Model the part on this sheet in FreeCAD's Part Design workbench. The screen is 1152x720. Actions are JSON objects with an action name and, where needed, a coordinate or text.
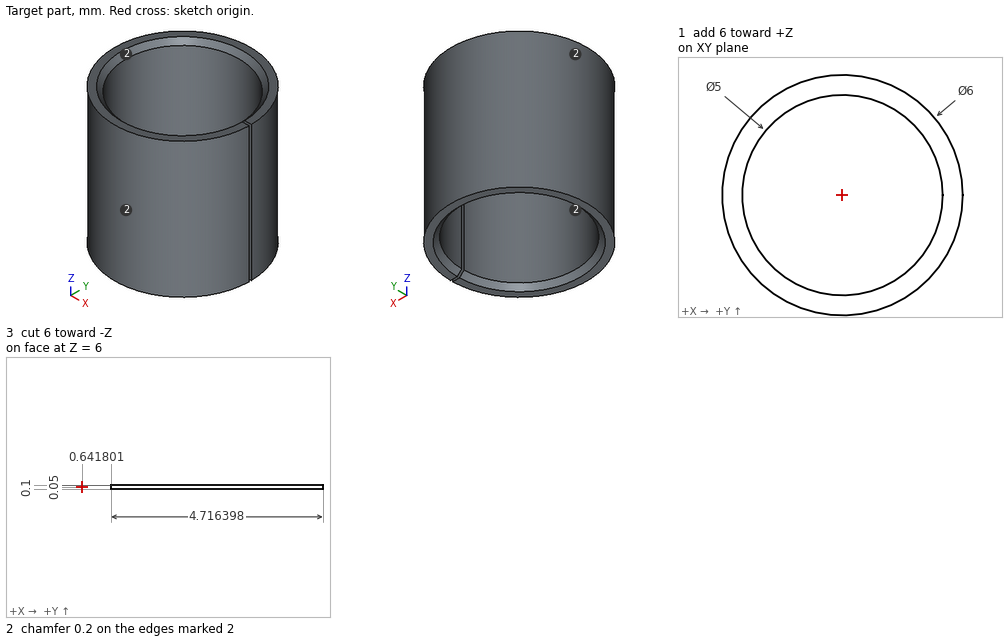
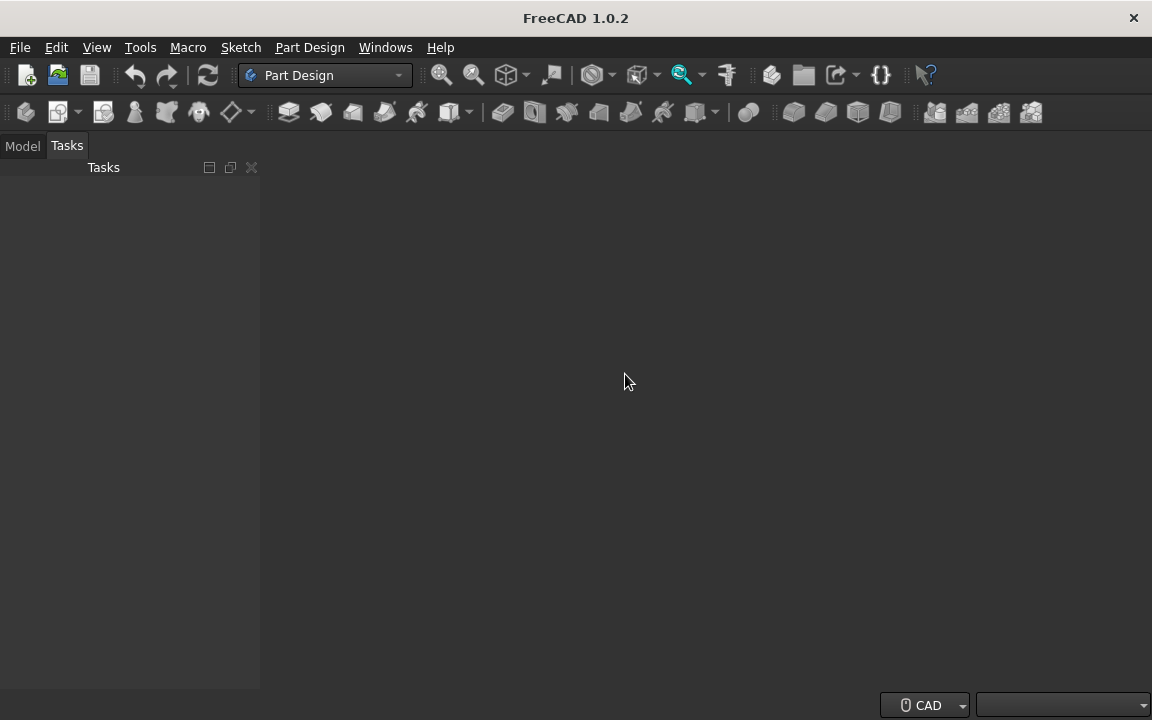
{"action": "left_click", "coordinate": [26, 76]}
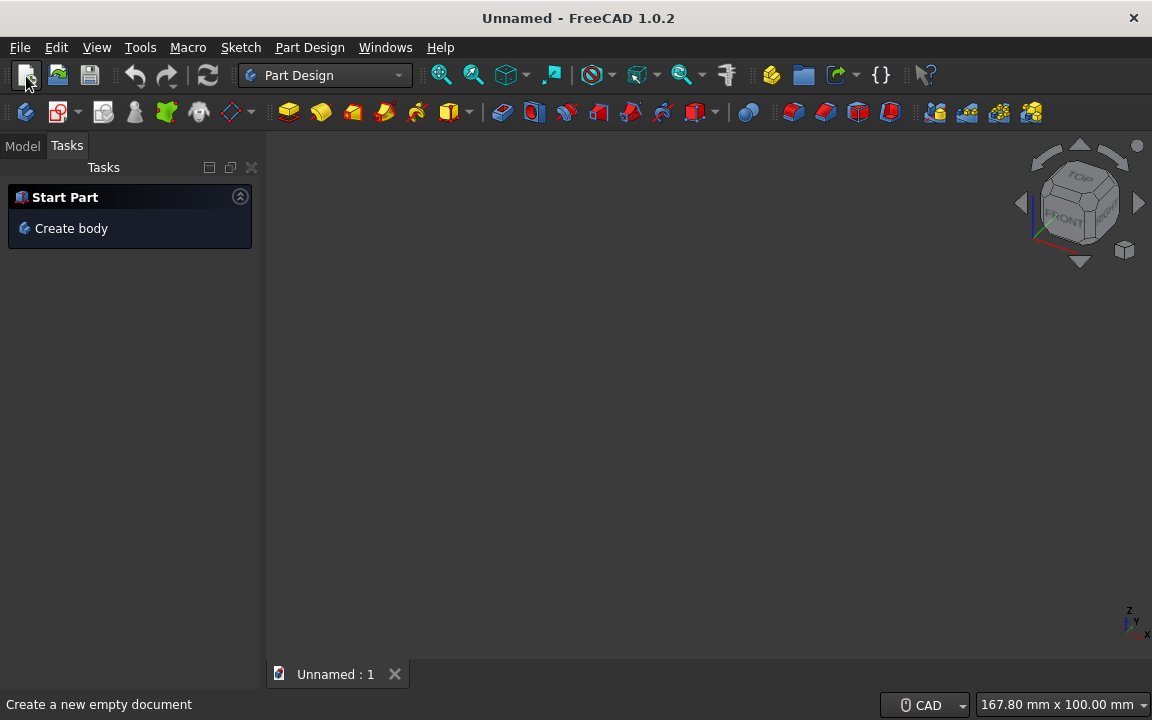
{"action": "left_click", "coordinate": [58, 112]}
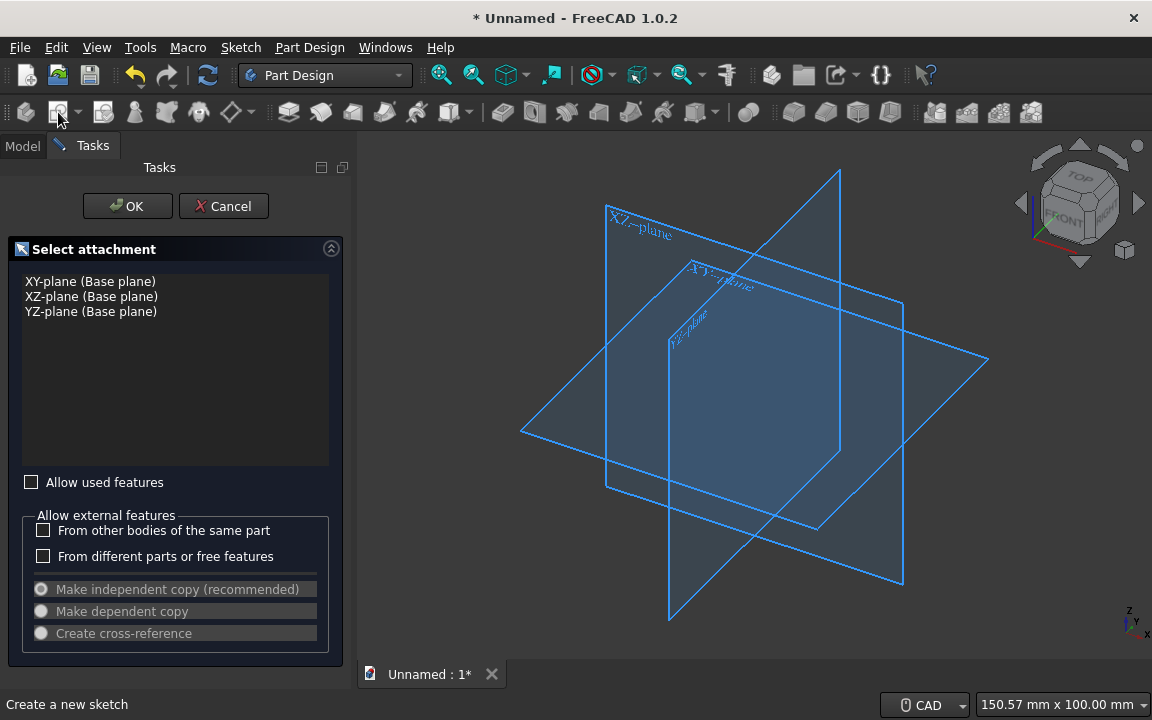
{"action": "left_click", "coordinate": [82, 282]}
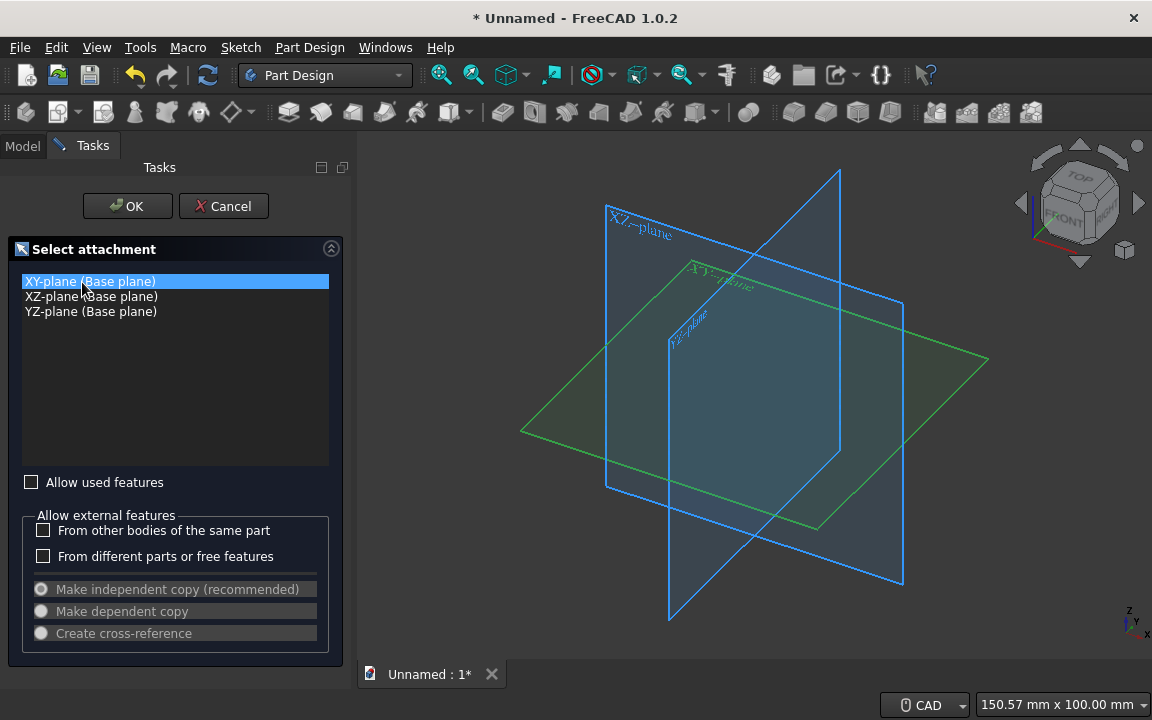
{"action": "left_click", "coordinate": [128, 206]}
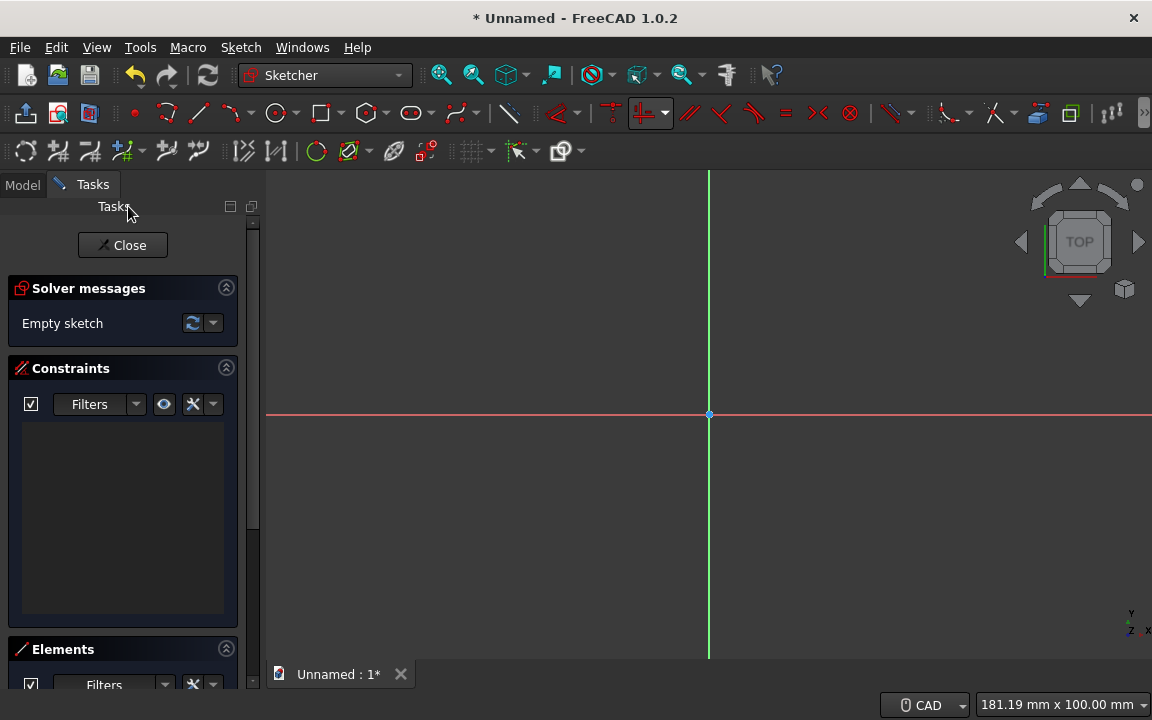
{"action": "scroll", "coordinate": [716, 414], "scroll_direction": "up", "scroll_amount": 12}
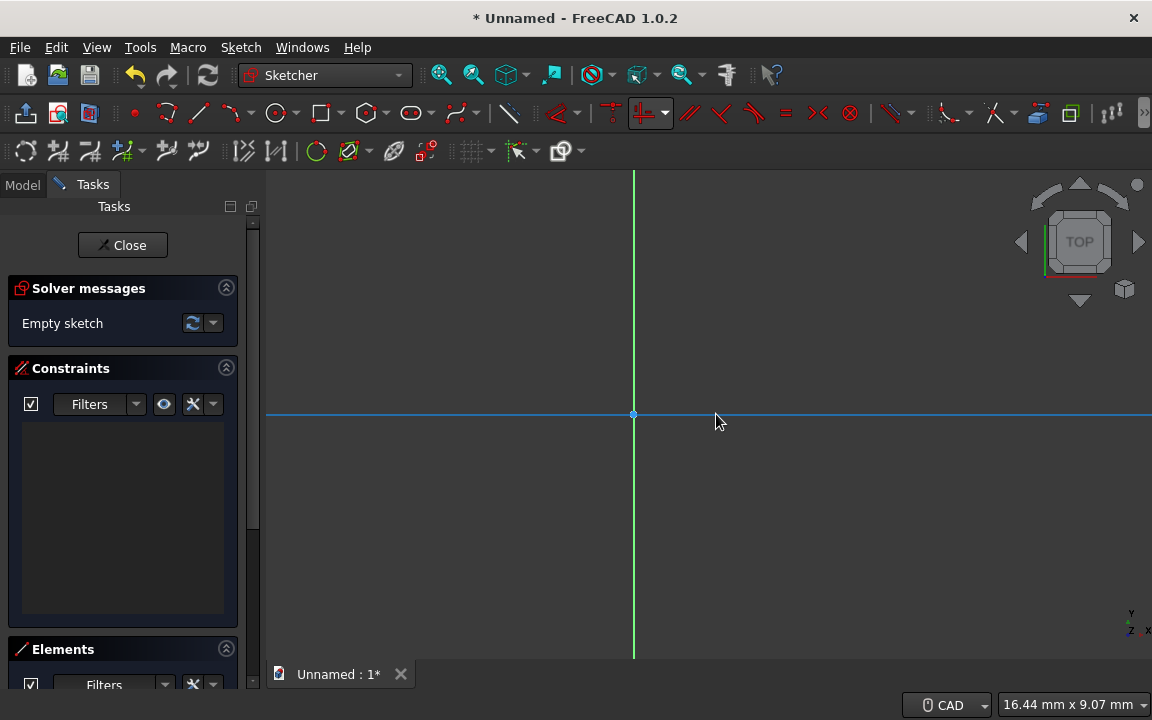
{"action": "left_click", "coordinate": [276, 114]}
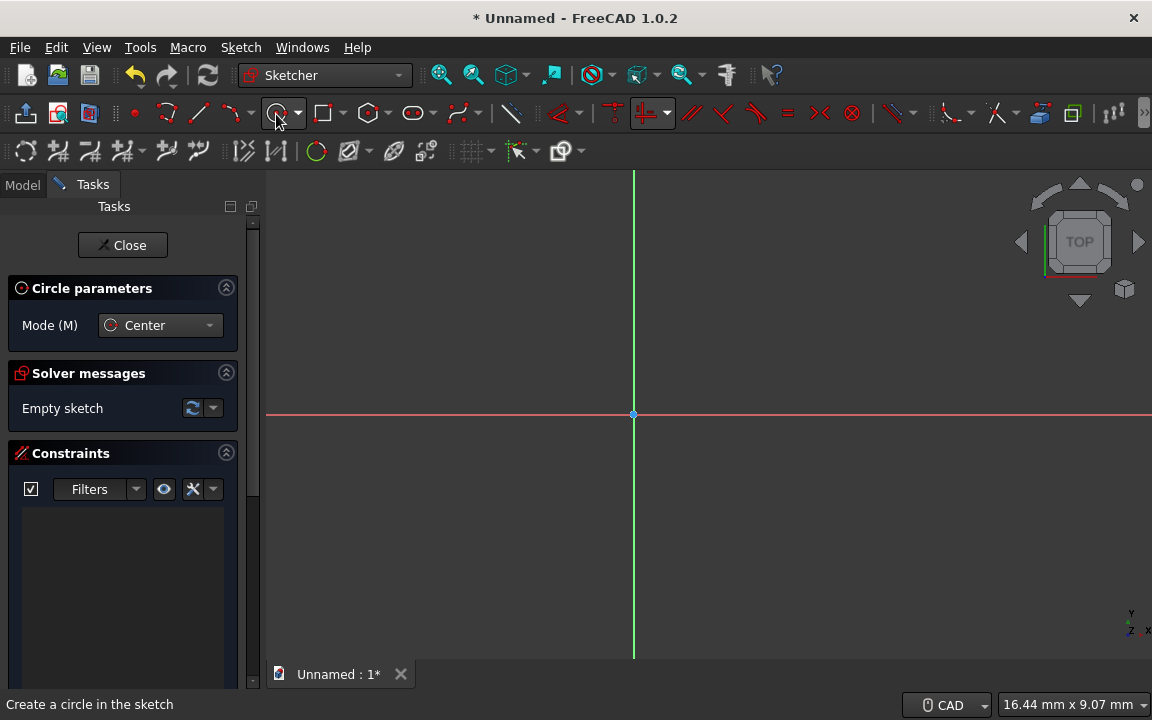
{"action": "left_click", "coordinate": [634, 414]}
{"action": "mouse_move", "coordinate": [748, 300]}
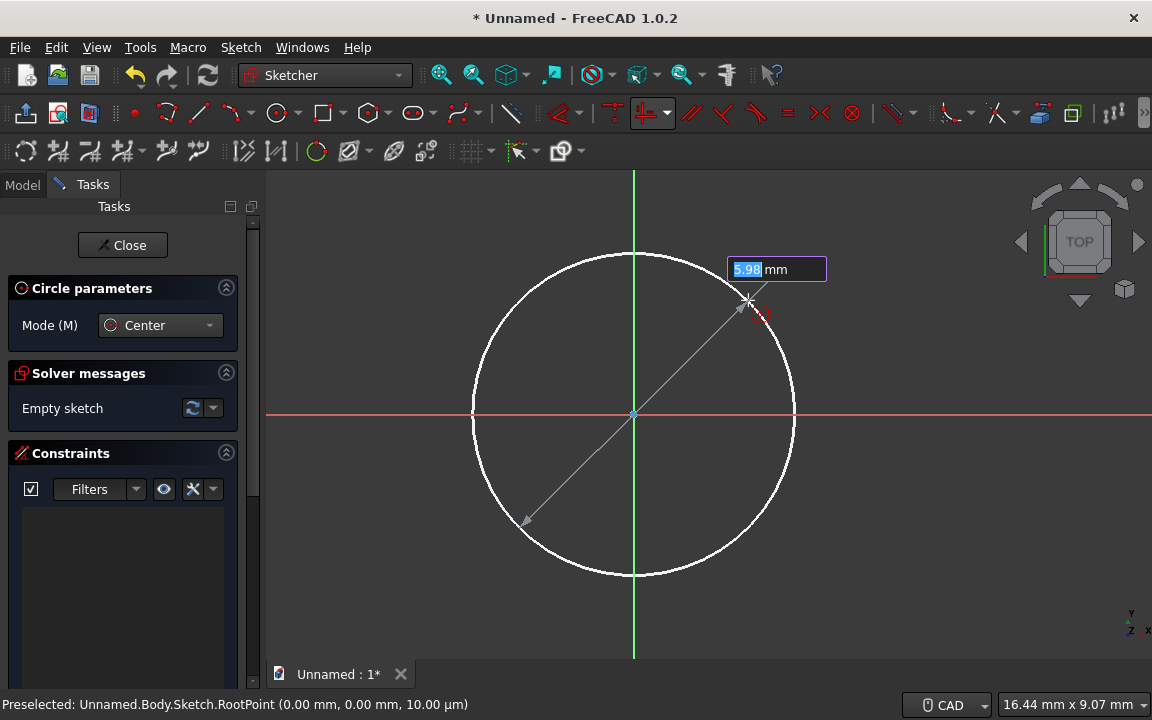
{"action": "type", "text": "6"}
{"action": "key", "text": "Return"}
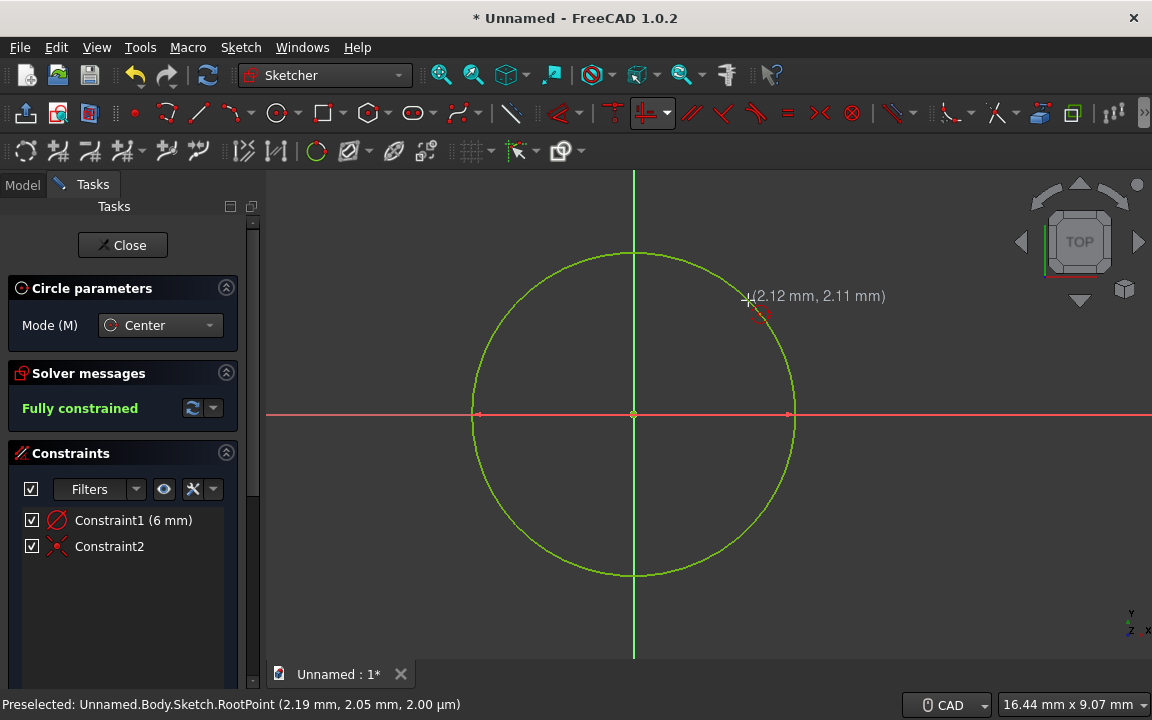
{"action": "left_click", "coordinate": [634, 414]}
{"action": "mouse_move", "coordinate": [729, 319]}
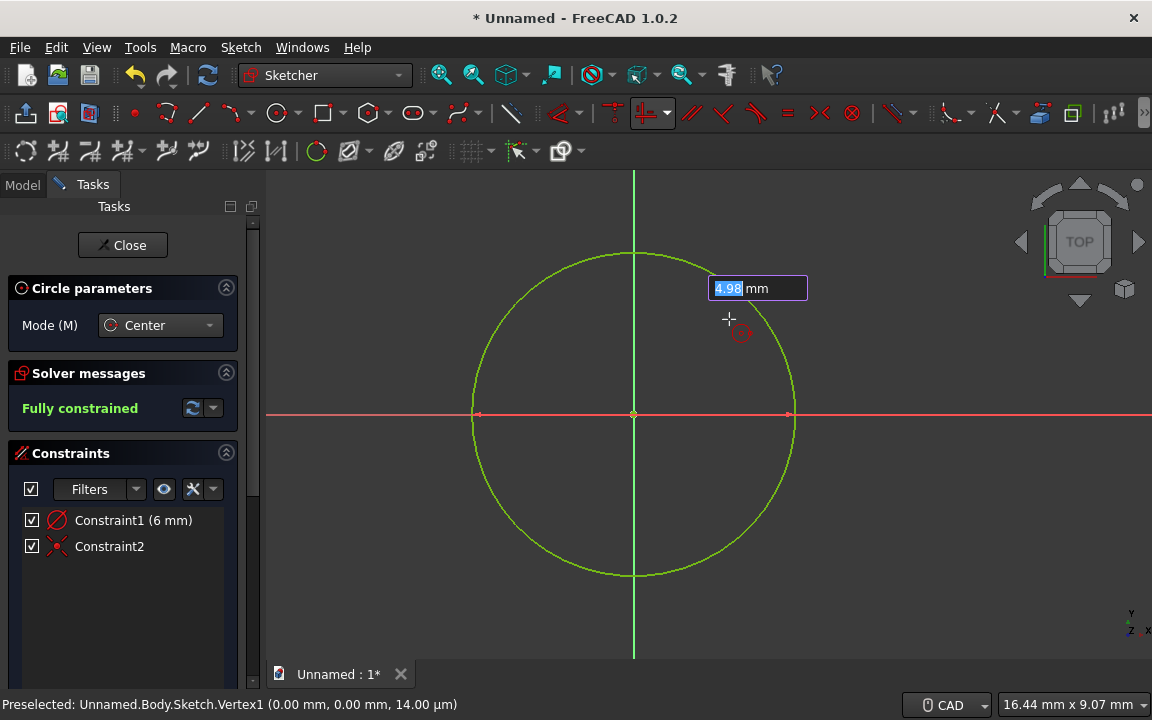
{"action": "type", "text": "5"}
{"action": "key", "text": "Return"}
{"action": "key", "text": "Escape"}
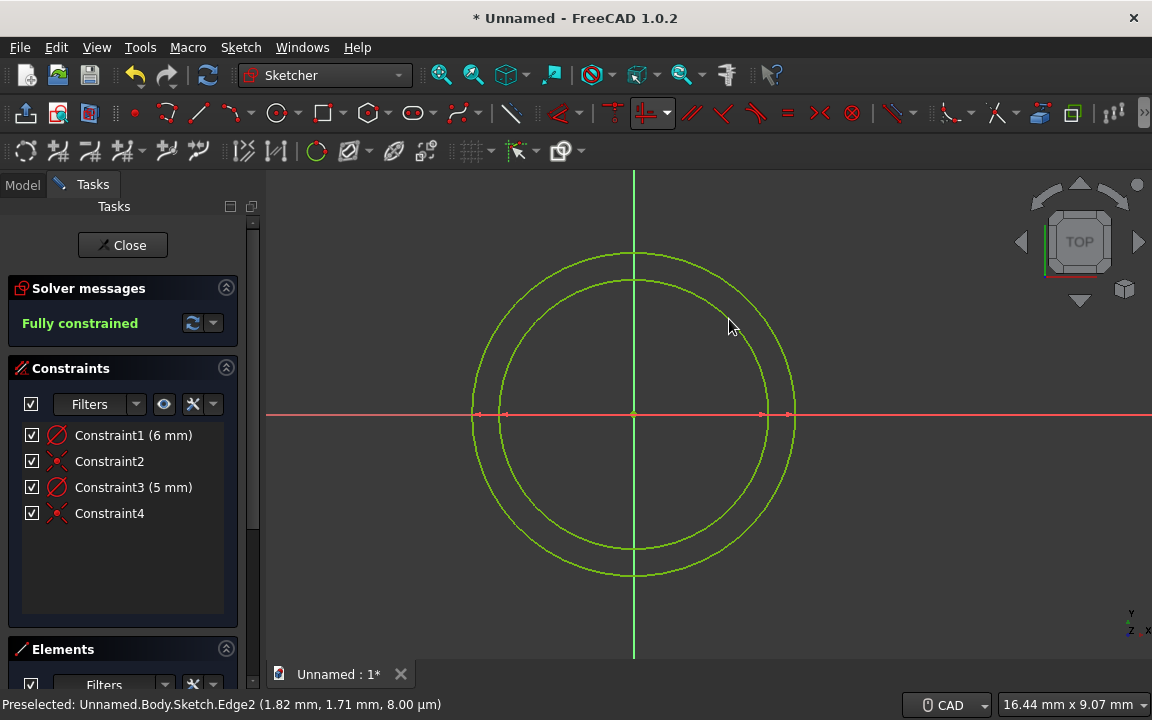
{"action": "left_click", "coordinate": [123, 245]}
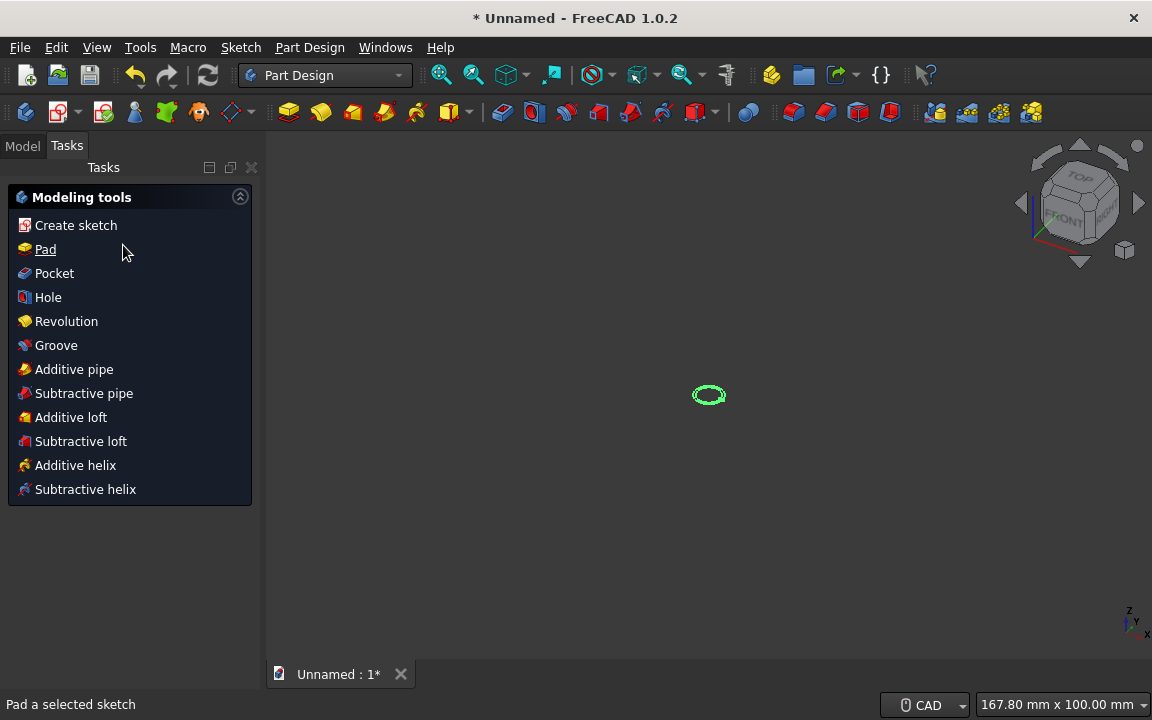
{"action": "left_click", "coordinate": [290, 112]}